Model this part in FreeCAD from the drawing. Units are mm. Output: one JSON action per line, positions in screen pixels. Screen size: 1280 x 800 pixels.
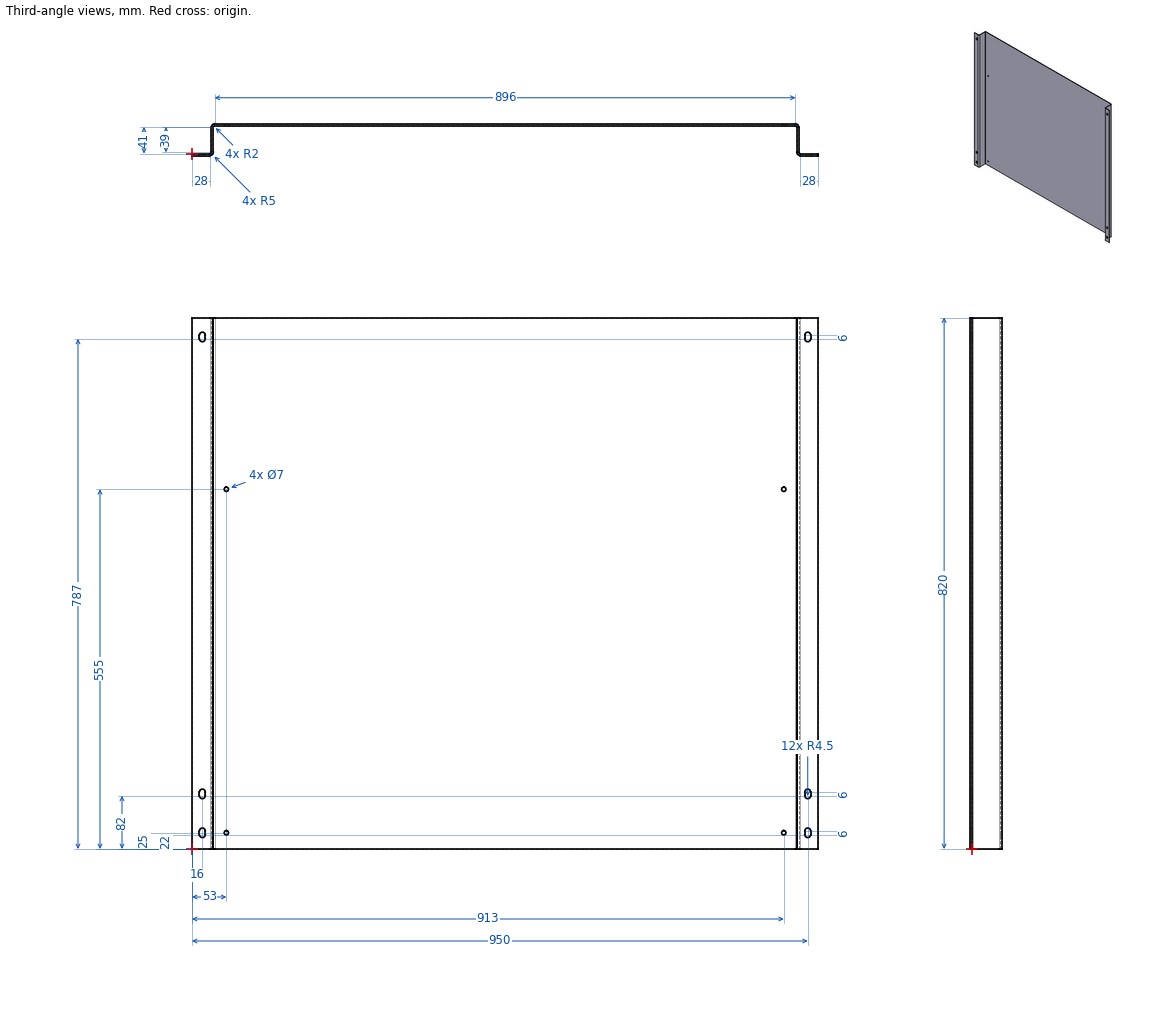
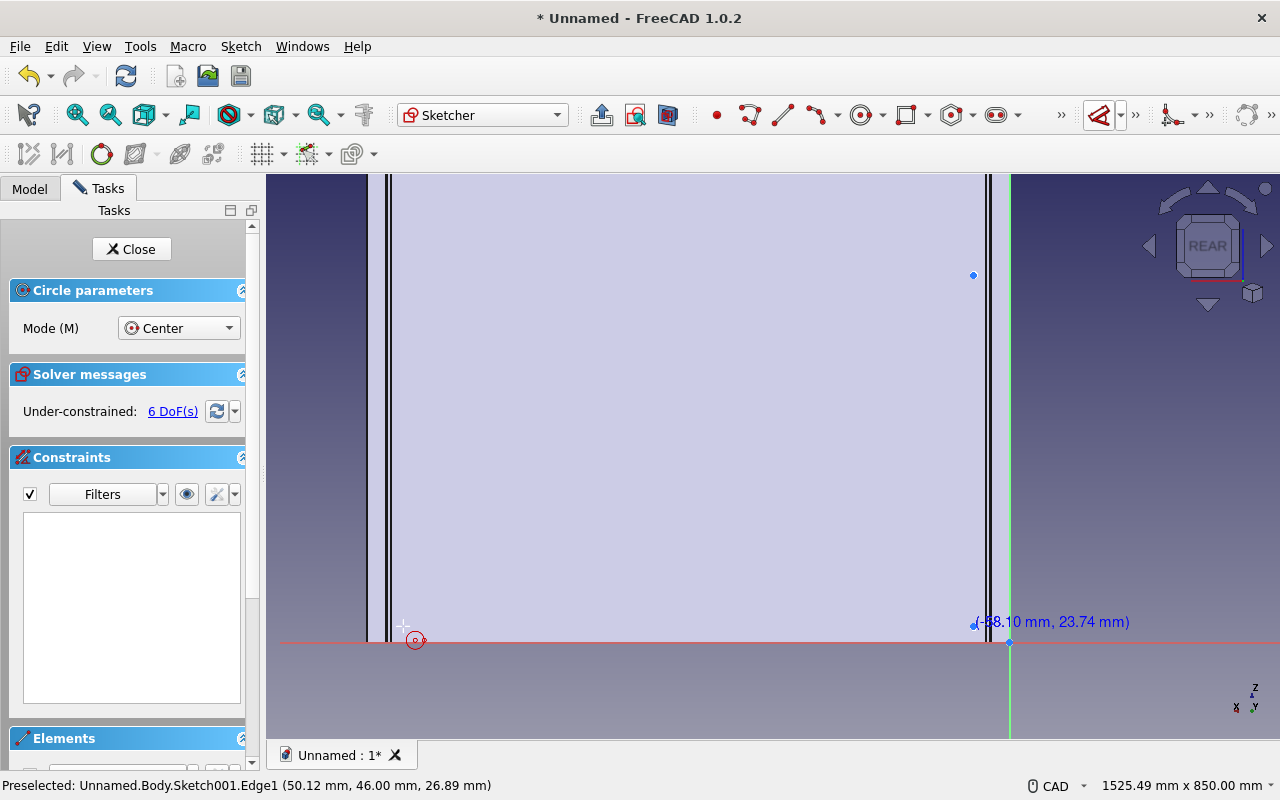
{"action": "left_click", "coordinate": [403, 626]}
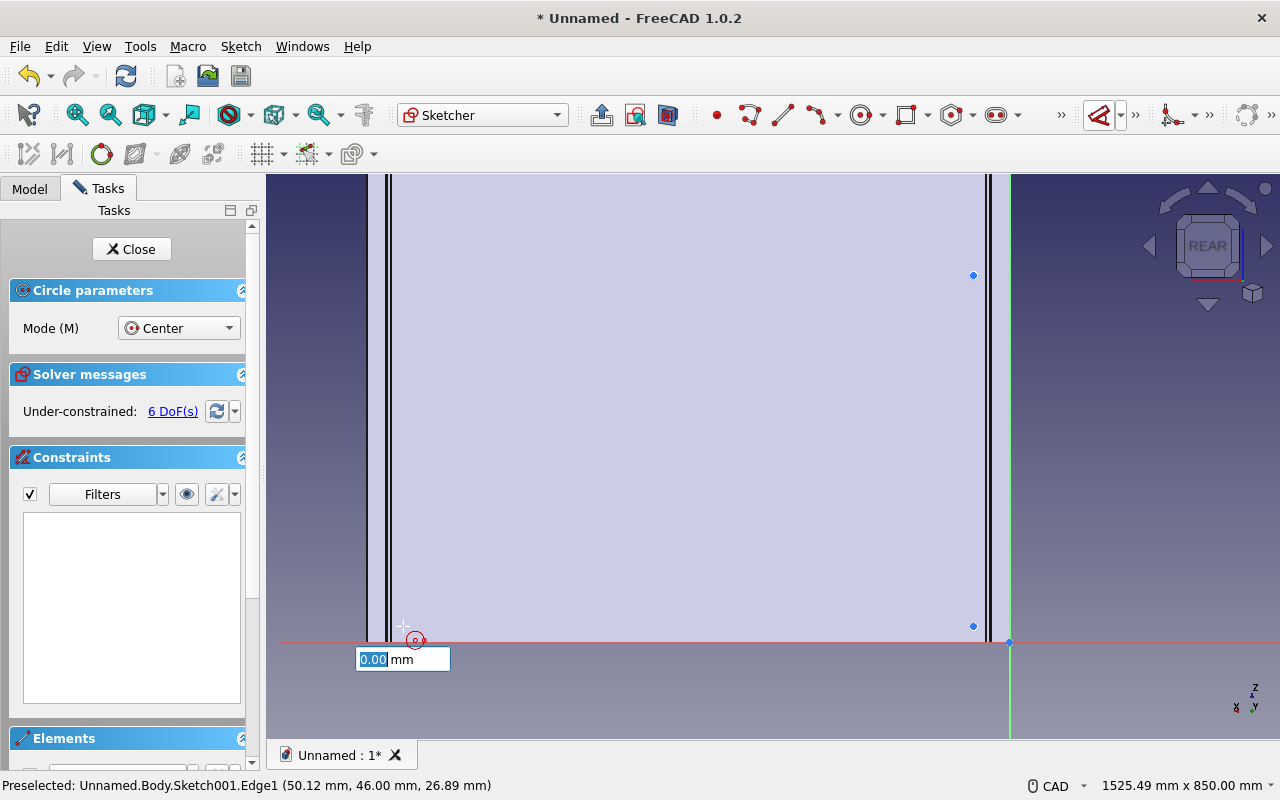
{"action": "scroll", "coordinate": [404, 625], "scroll_direction": "up", "scroll_amount": 10}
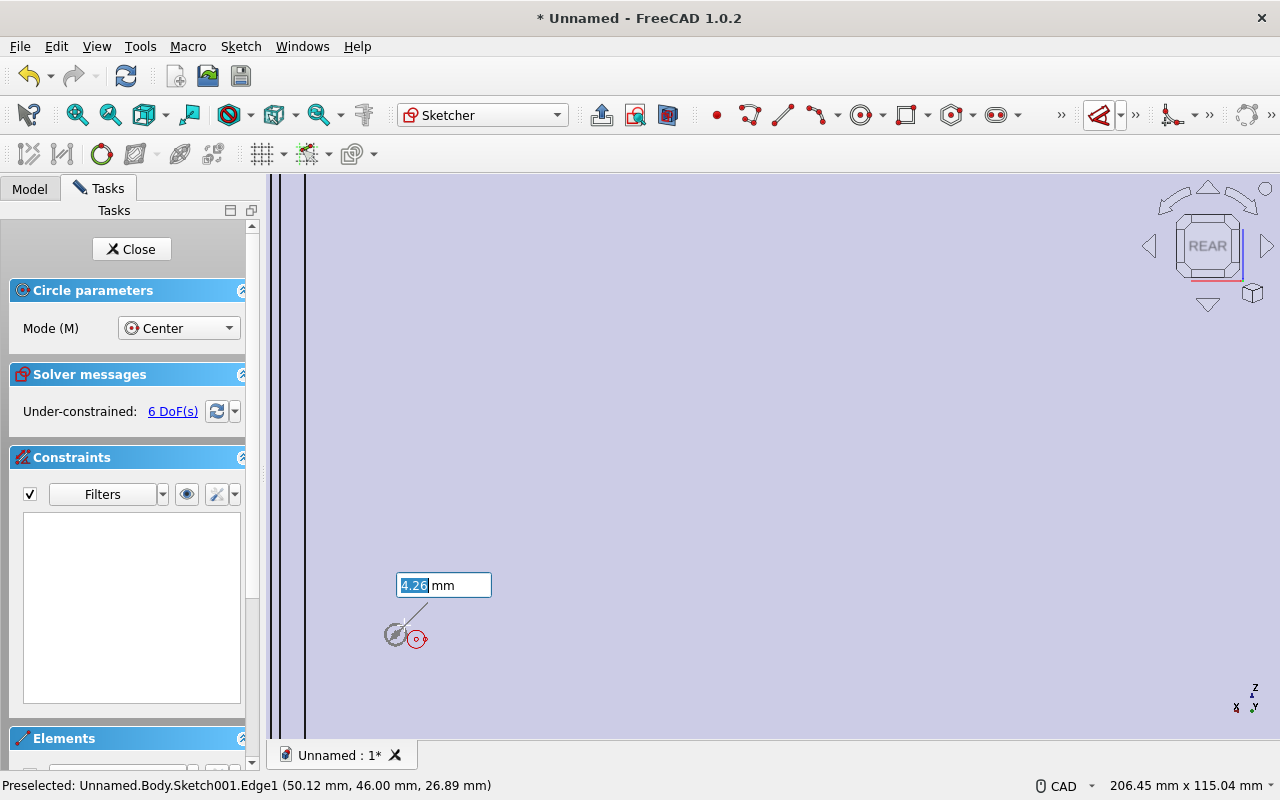
{"action": "left_click", "coordinate": [405, 616]}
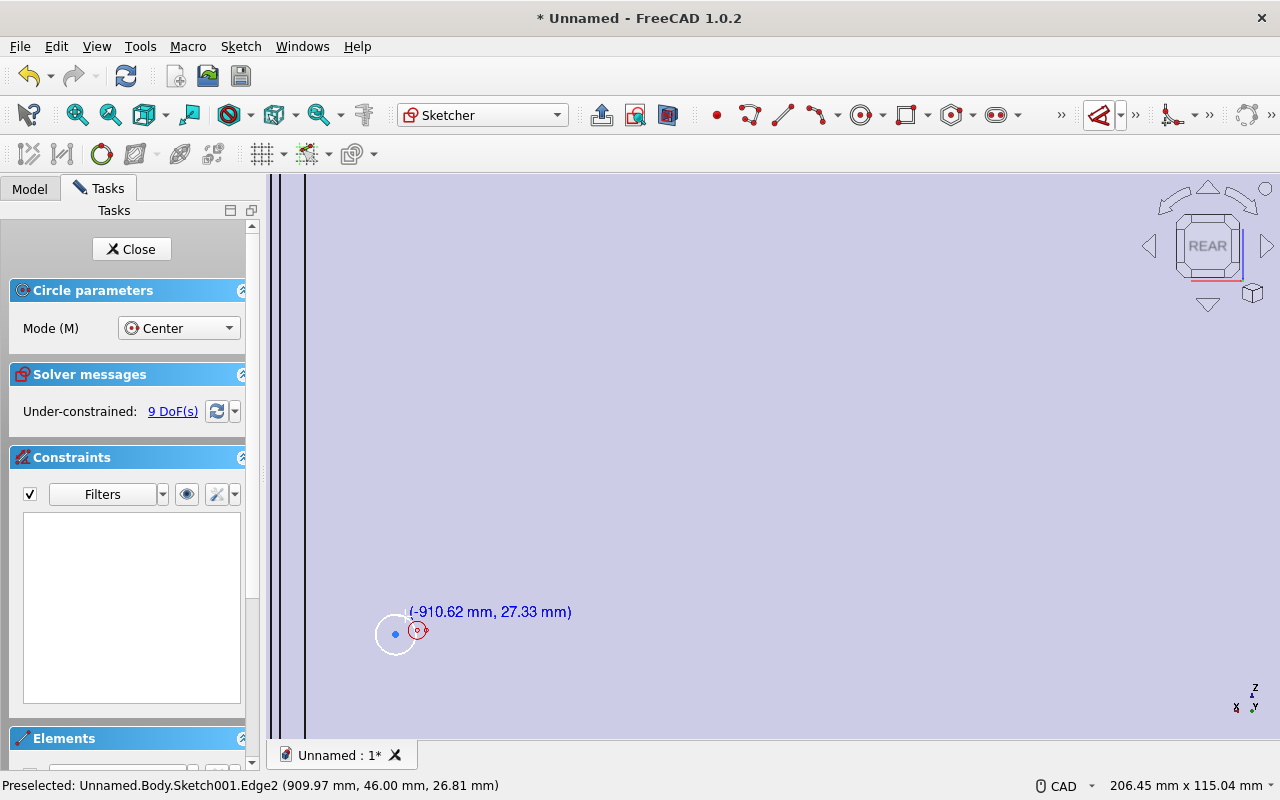
{"action": "scroll", "coordinate": [404, 625], "scroll_direction": "down", "scroll_amount": 10}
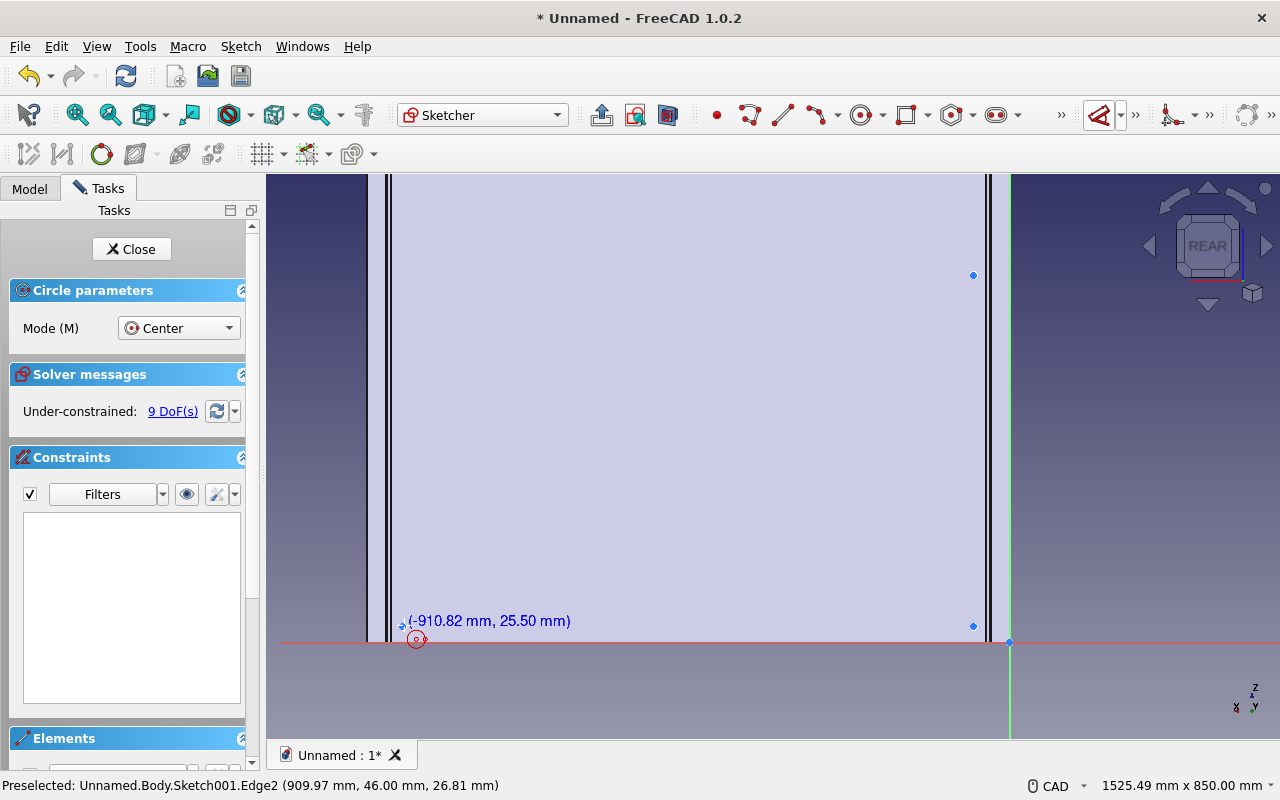
{"action": "scroll", "coordinate": [403, 274], "scroll_direction": "up", "scroll_amount": 12}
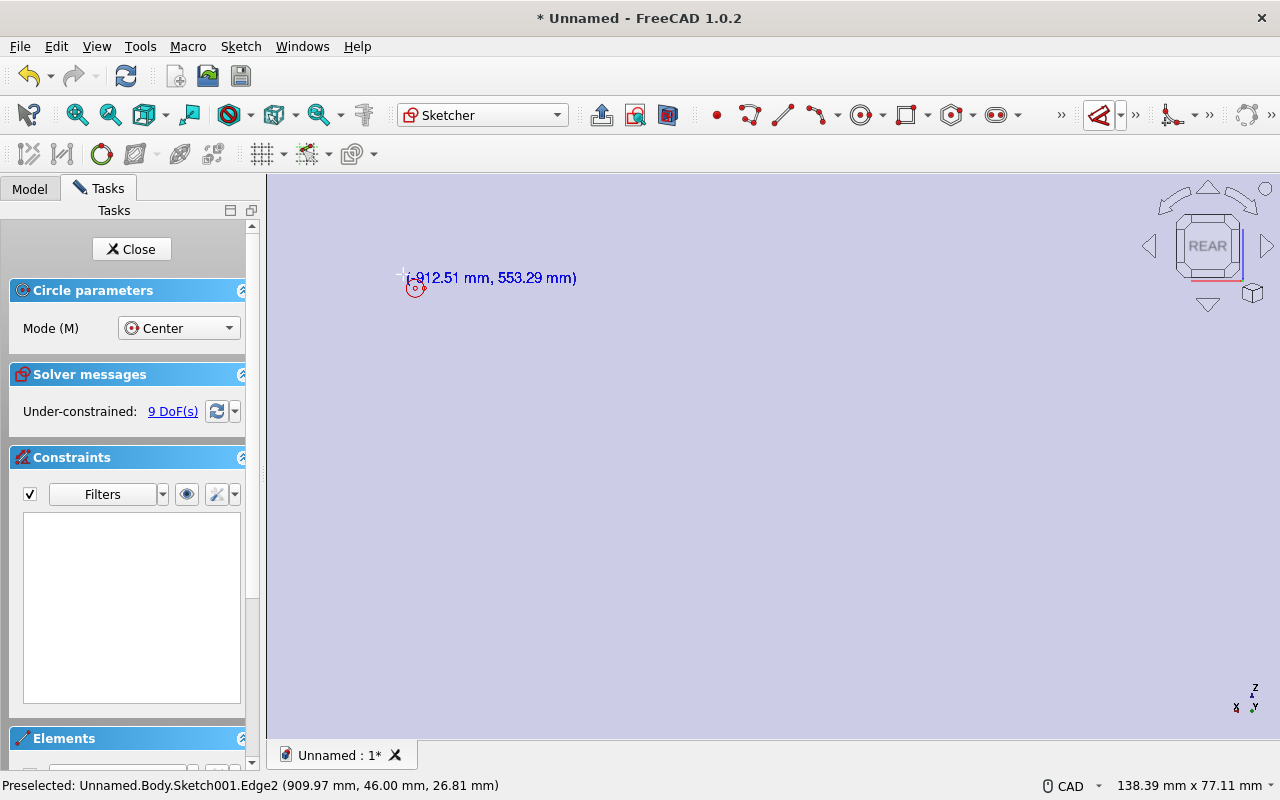
{"action": "scroll", "coordinate": [403, 273], "scroll_direction": "down", "scroll_amount": 12}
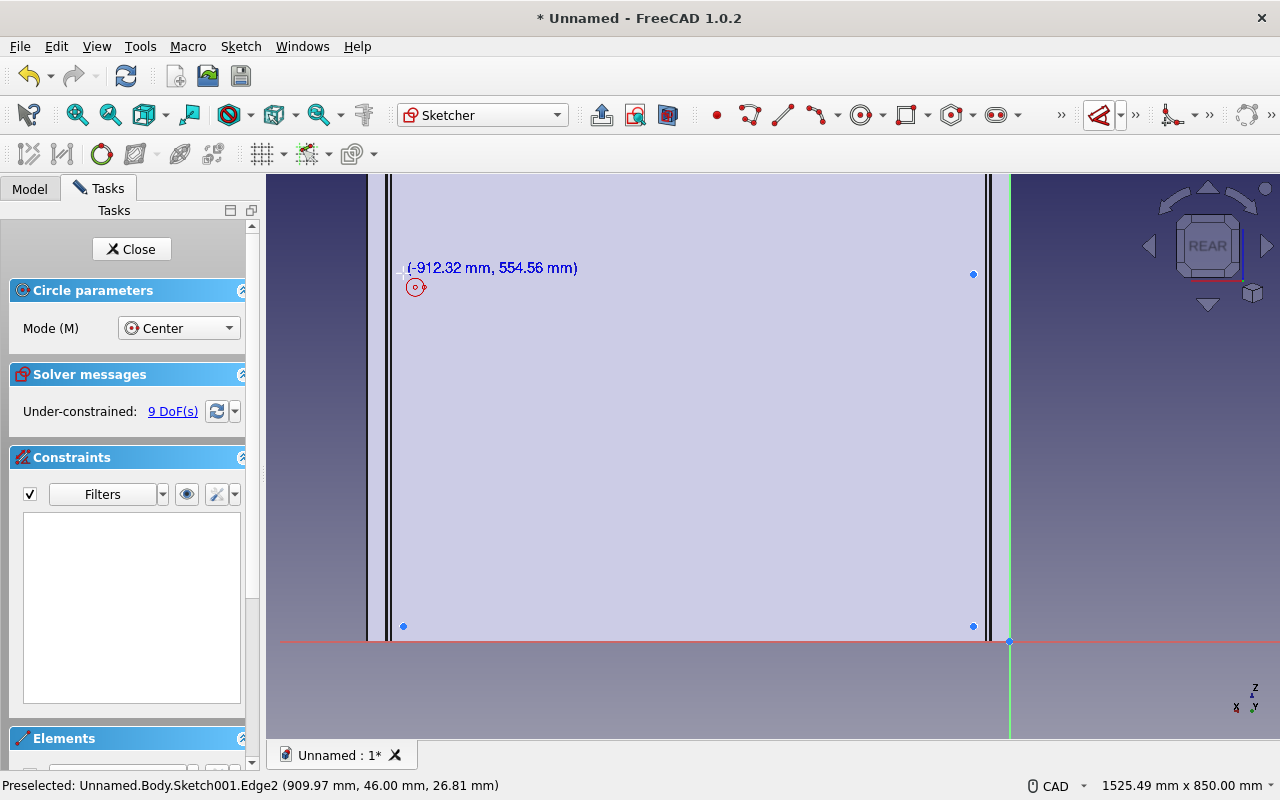
{"action": "left_click", "coordinate": [403, 273]}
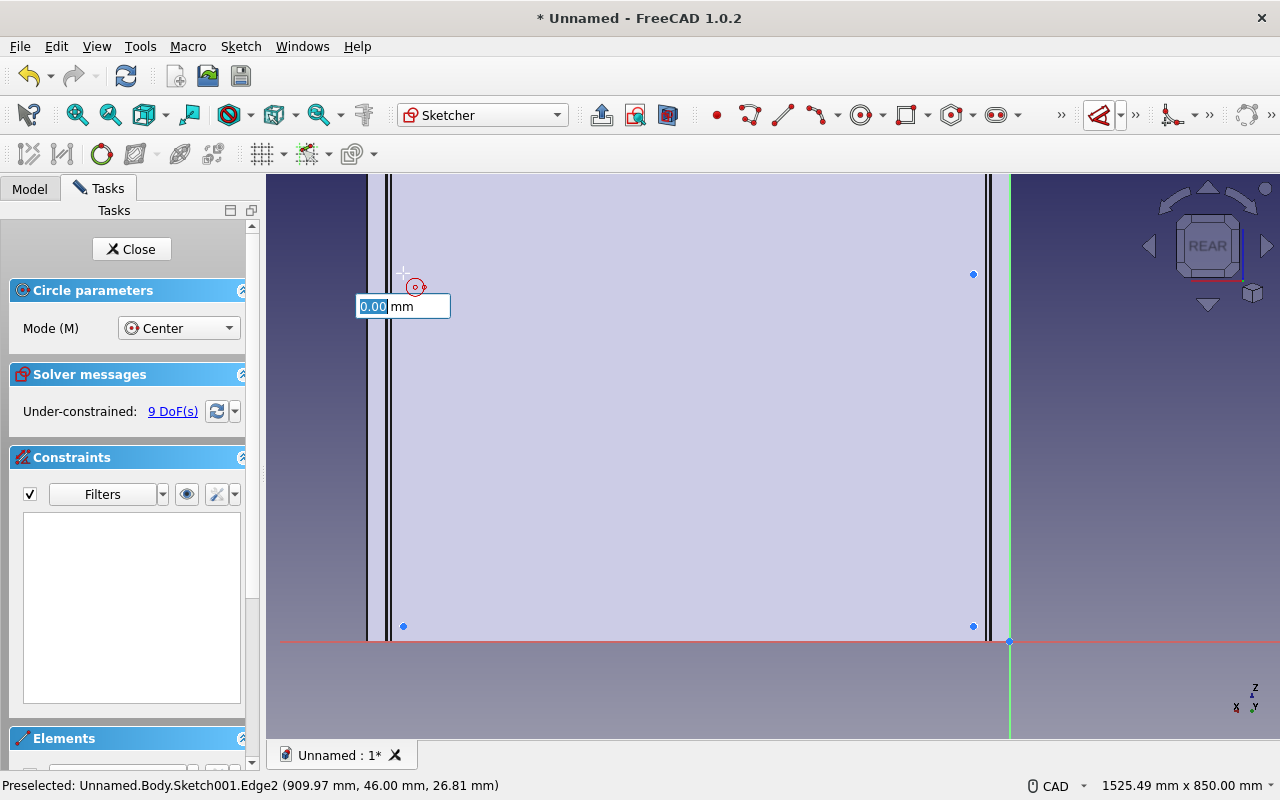
{"action": "scroll", "coordinate": [404, 271], "scroll_direction": "up", "scroll_amount": 10}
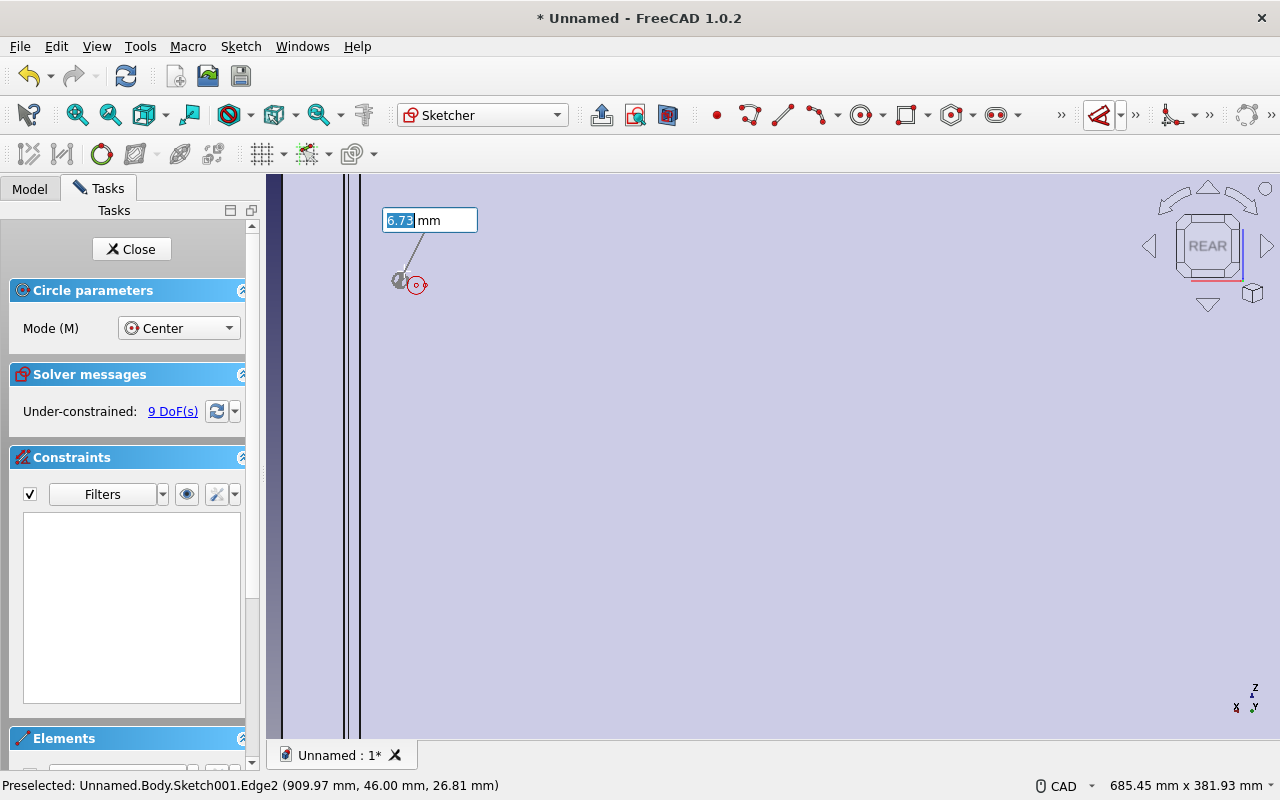
{"action": "left_click", "coordinate": [405, 272]}
{"action": "key", "text": "Escape"}